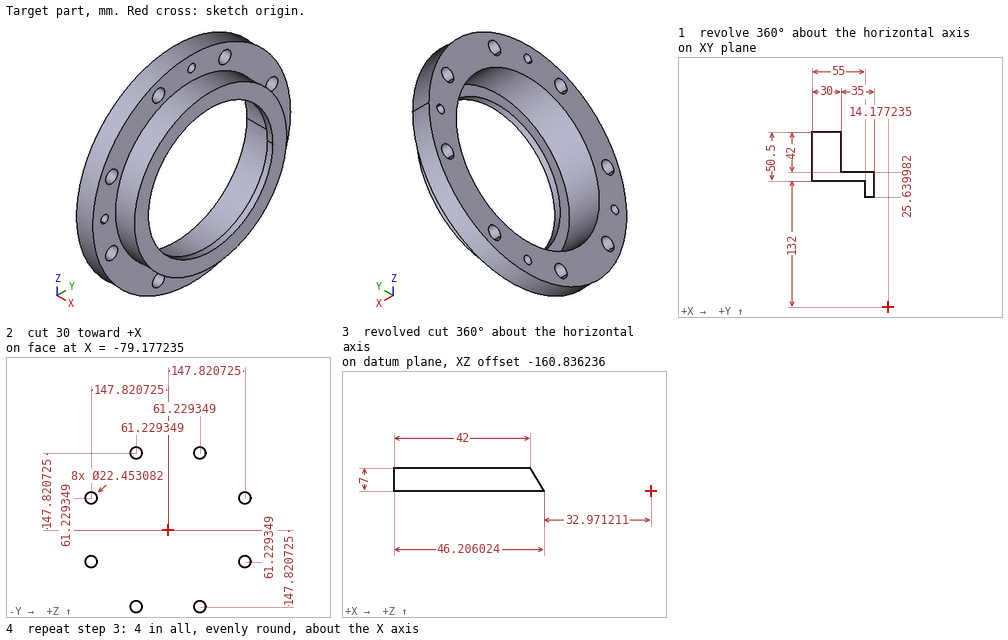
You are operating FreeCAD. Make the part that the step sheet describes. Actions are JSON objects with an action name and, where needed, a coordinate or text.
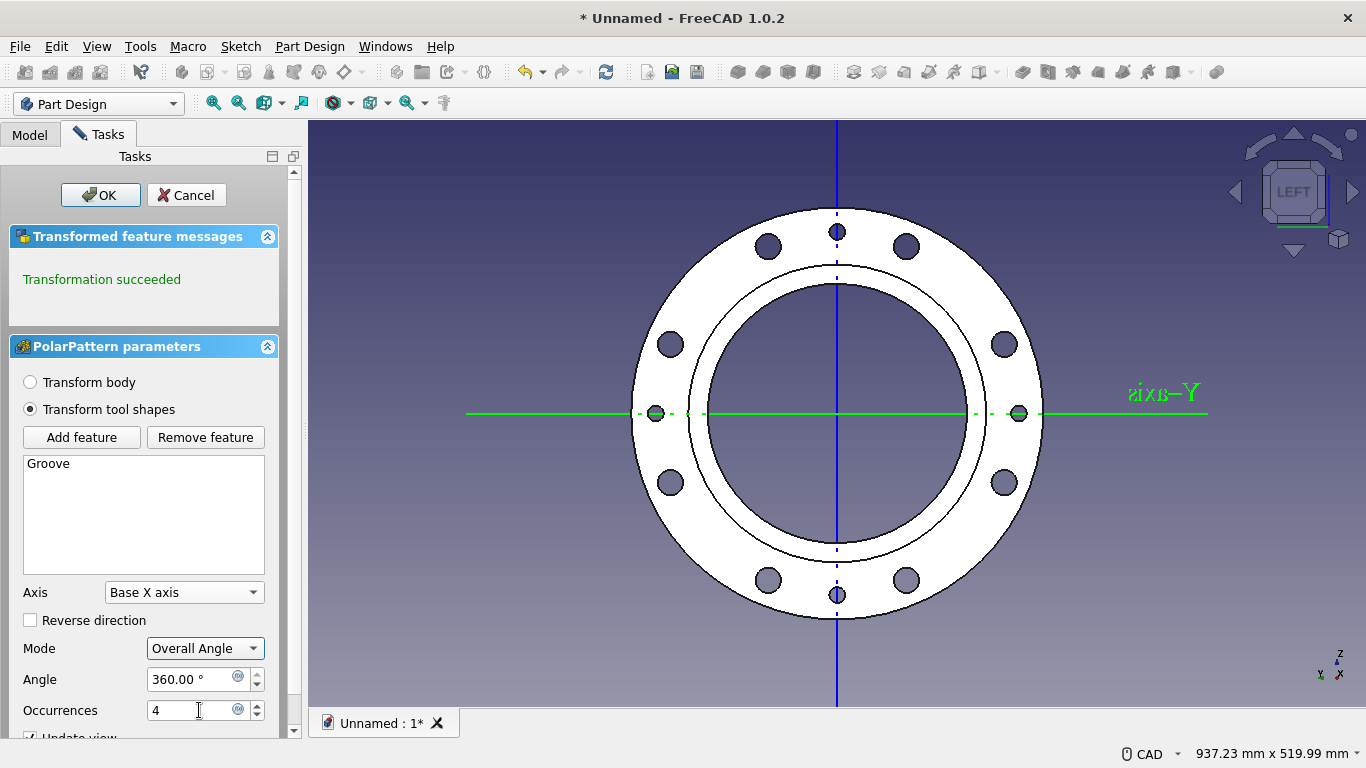
{"action": "left_click", "coordinate": [101, 195]}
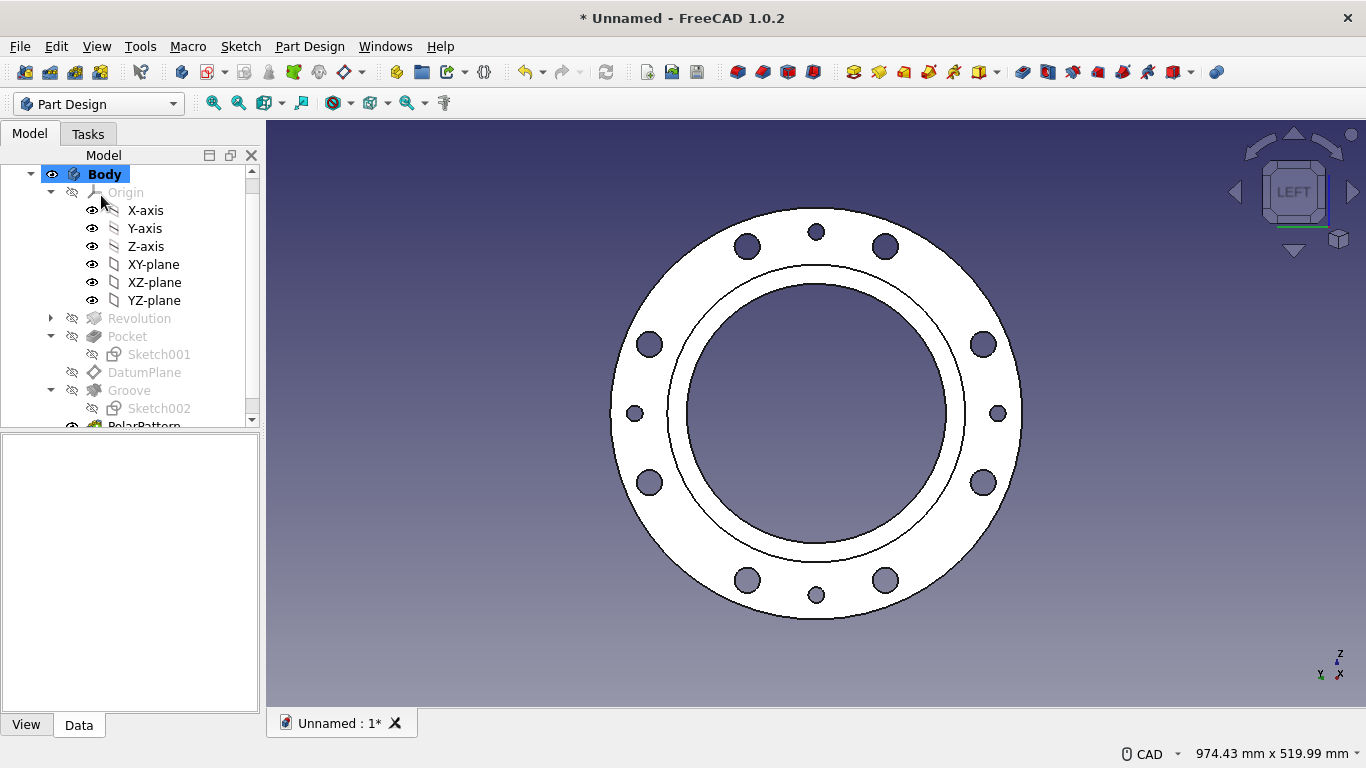
{"action": "key", "text": "0"}